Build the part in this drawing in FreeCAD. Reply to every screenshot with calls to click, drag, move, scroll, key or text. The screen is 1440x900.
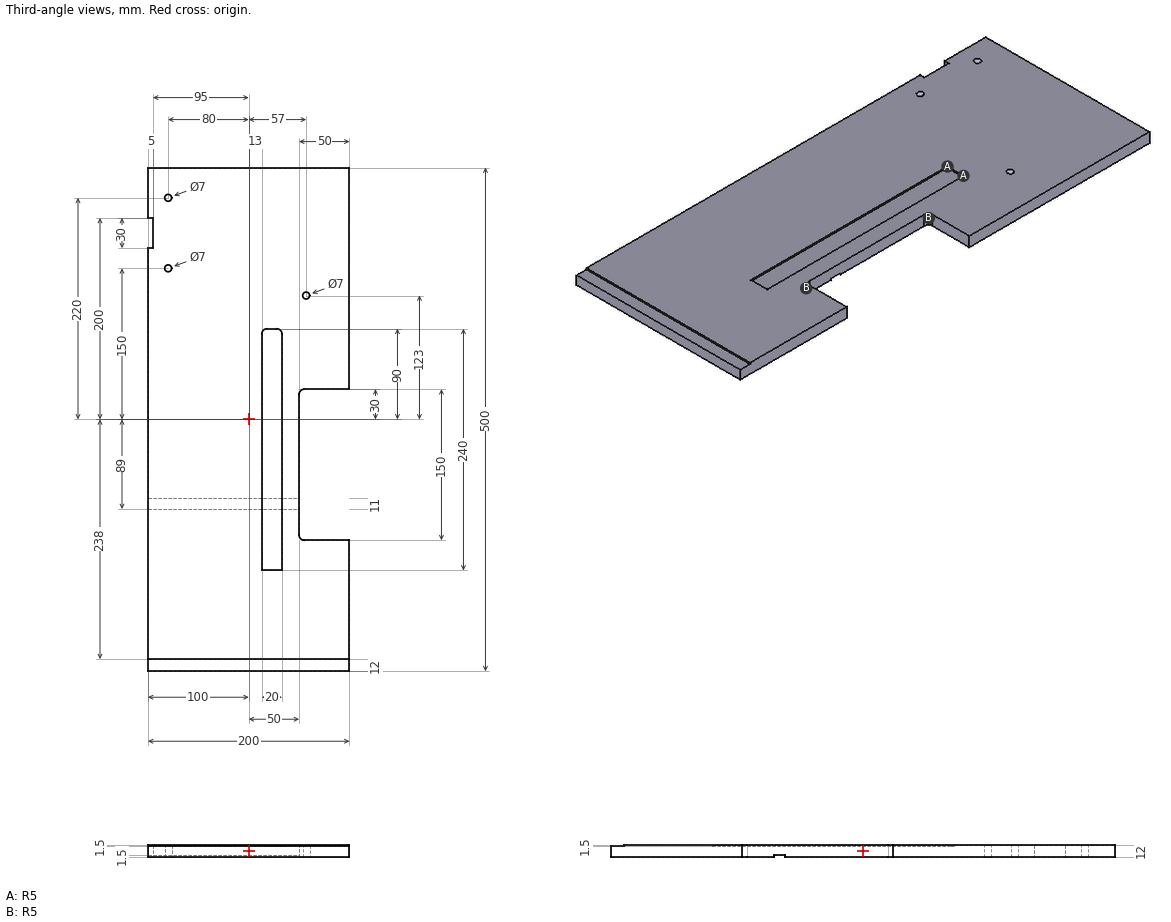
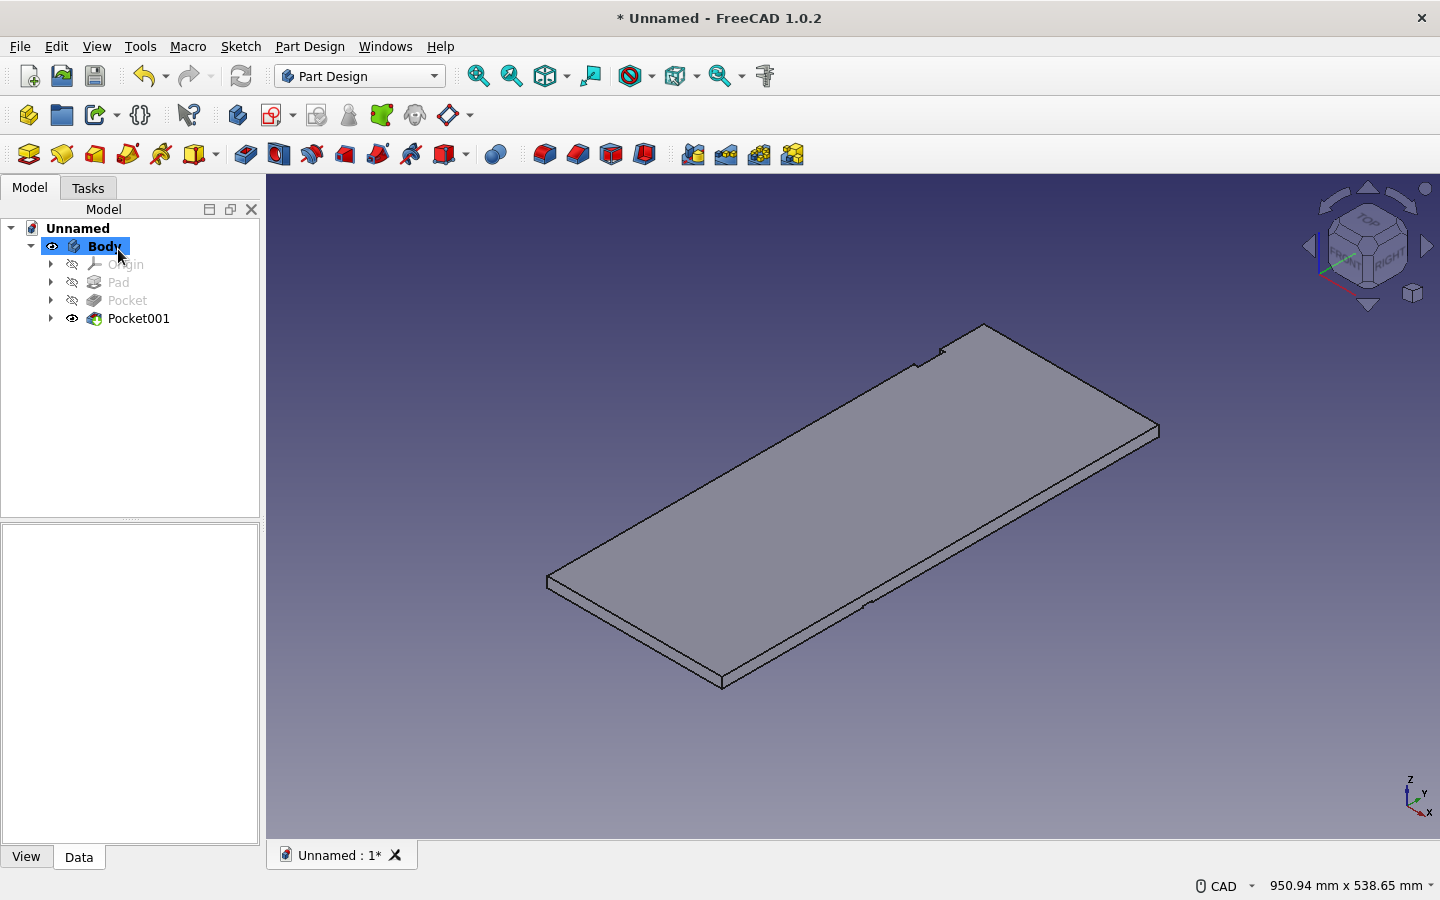
click(915, 463)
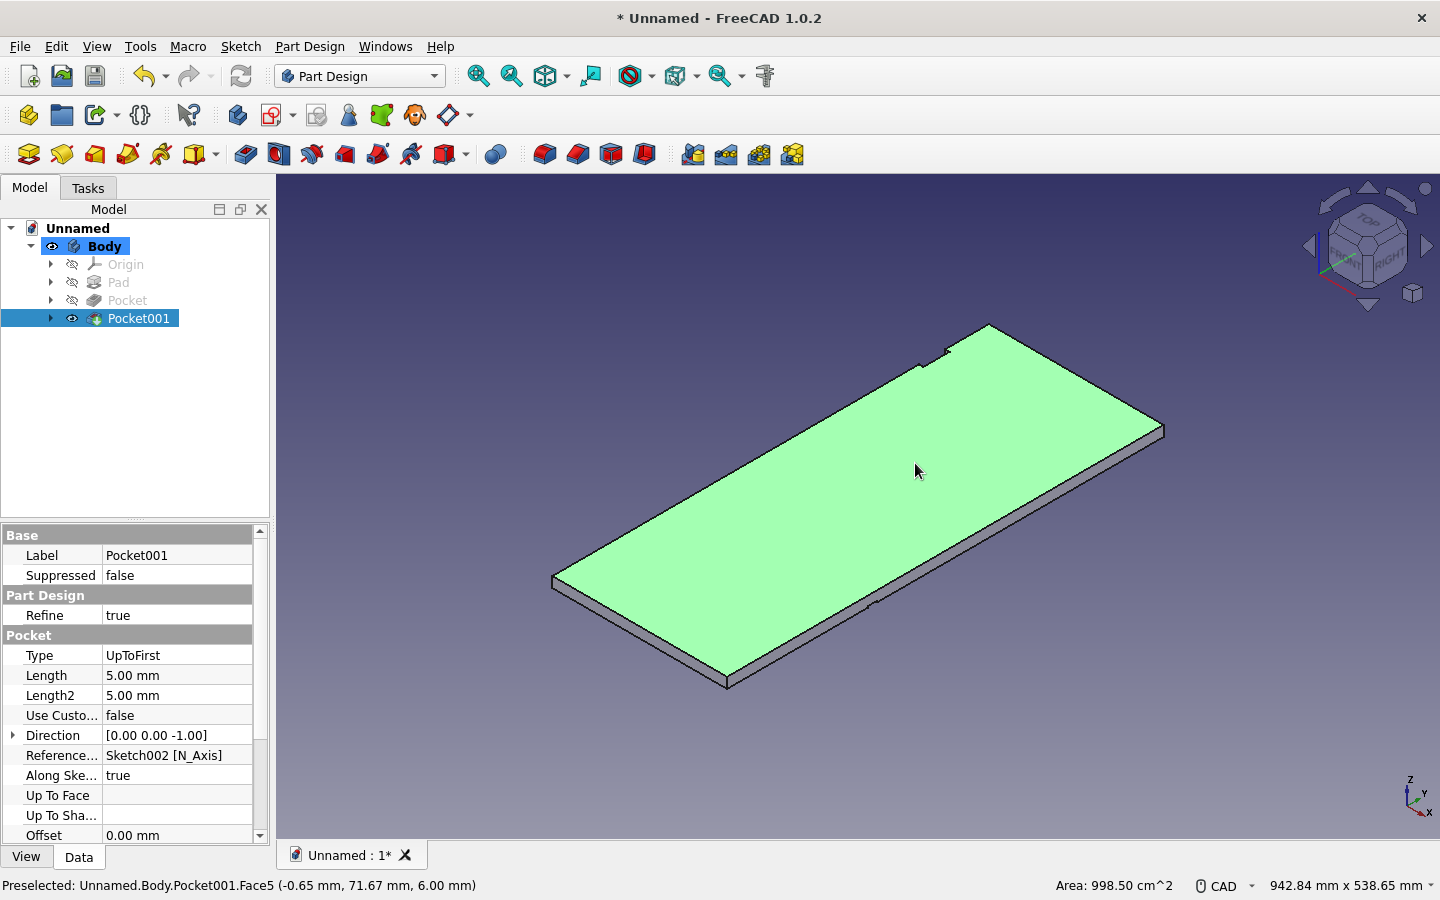
click(270, 116)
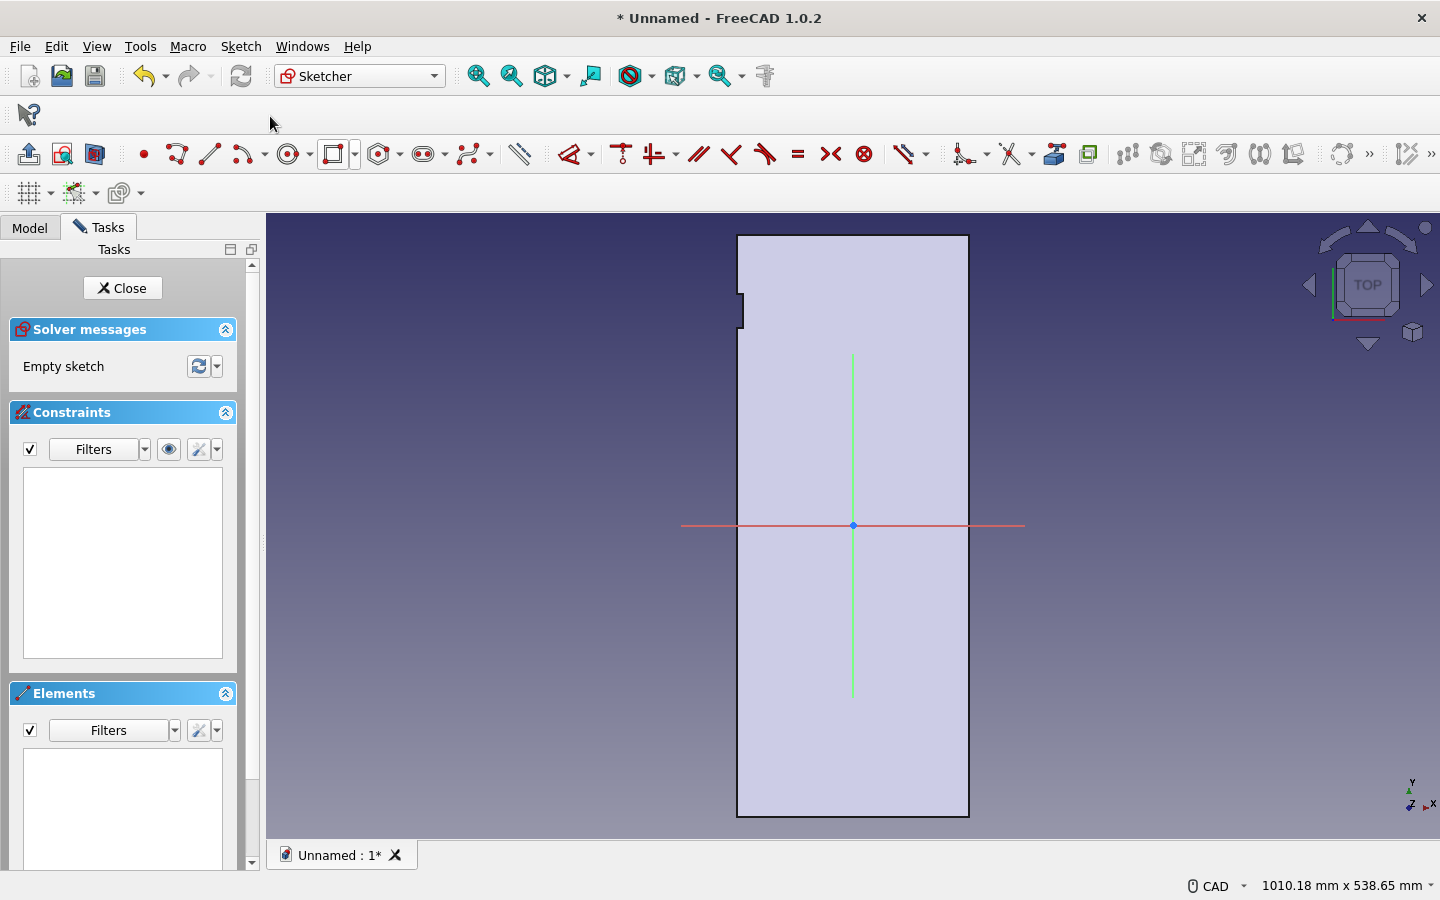
scroll(759, 257, up, 15)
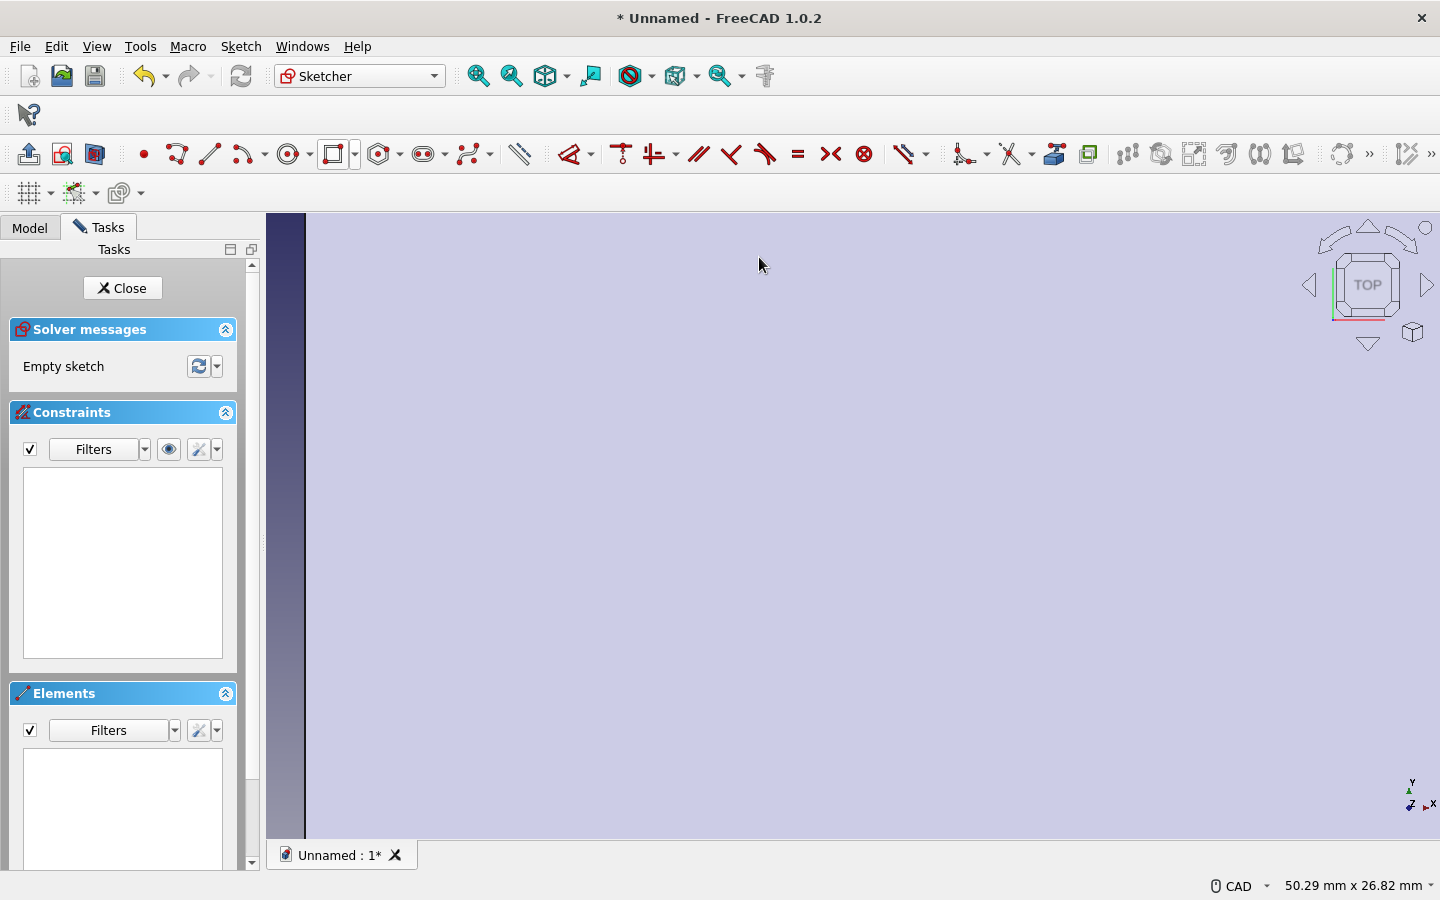
scroll(764, 522, up, 5)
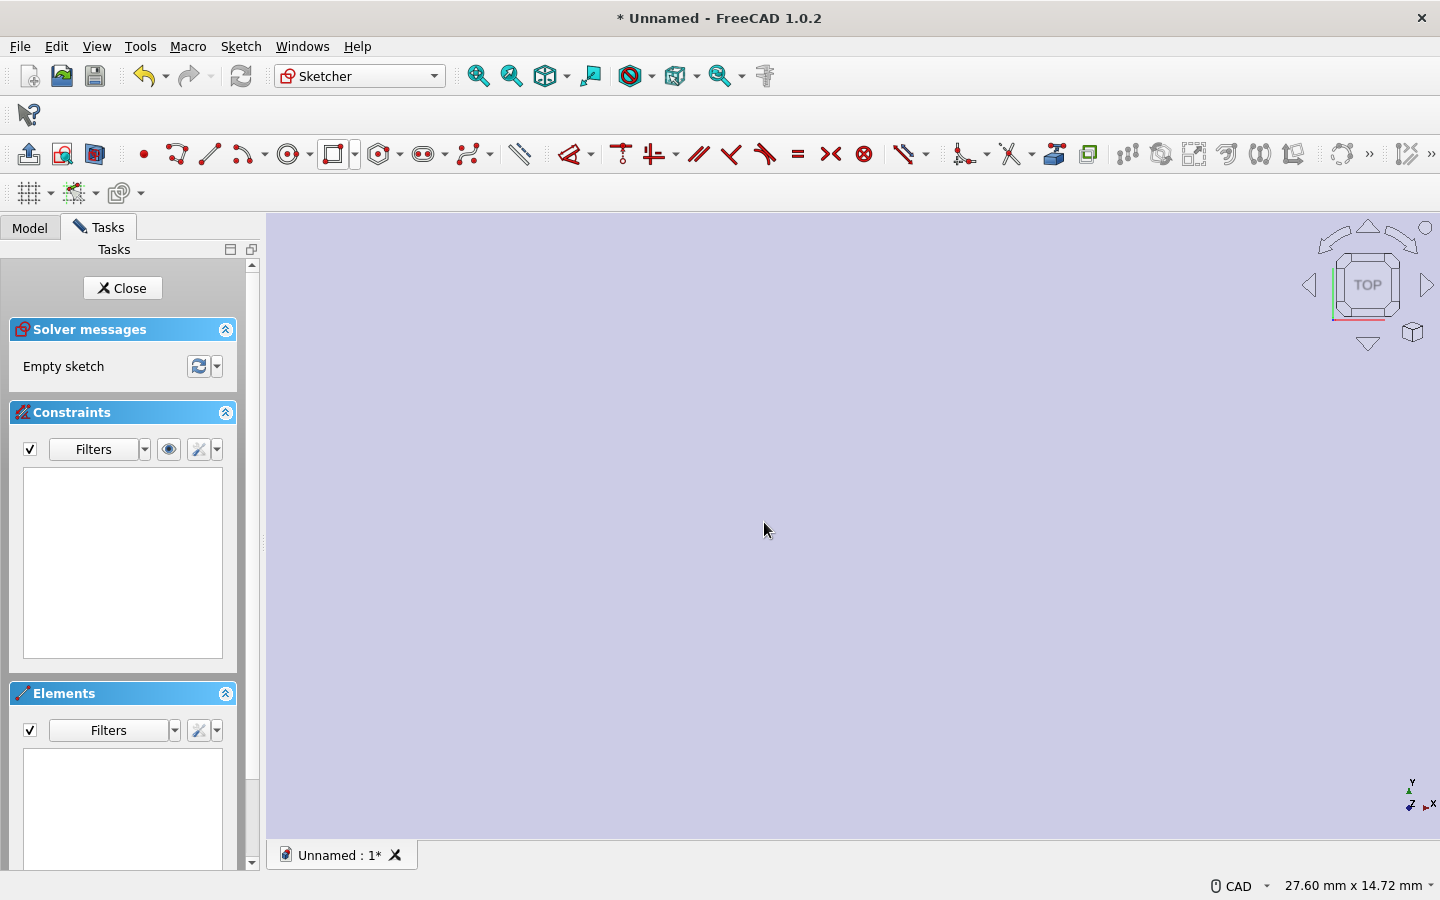
click(288, 154)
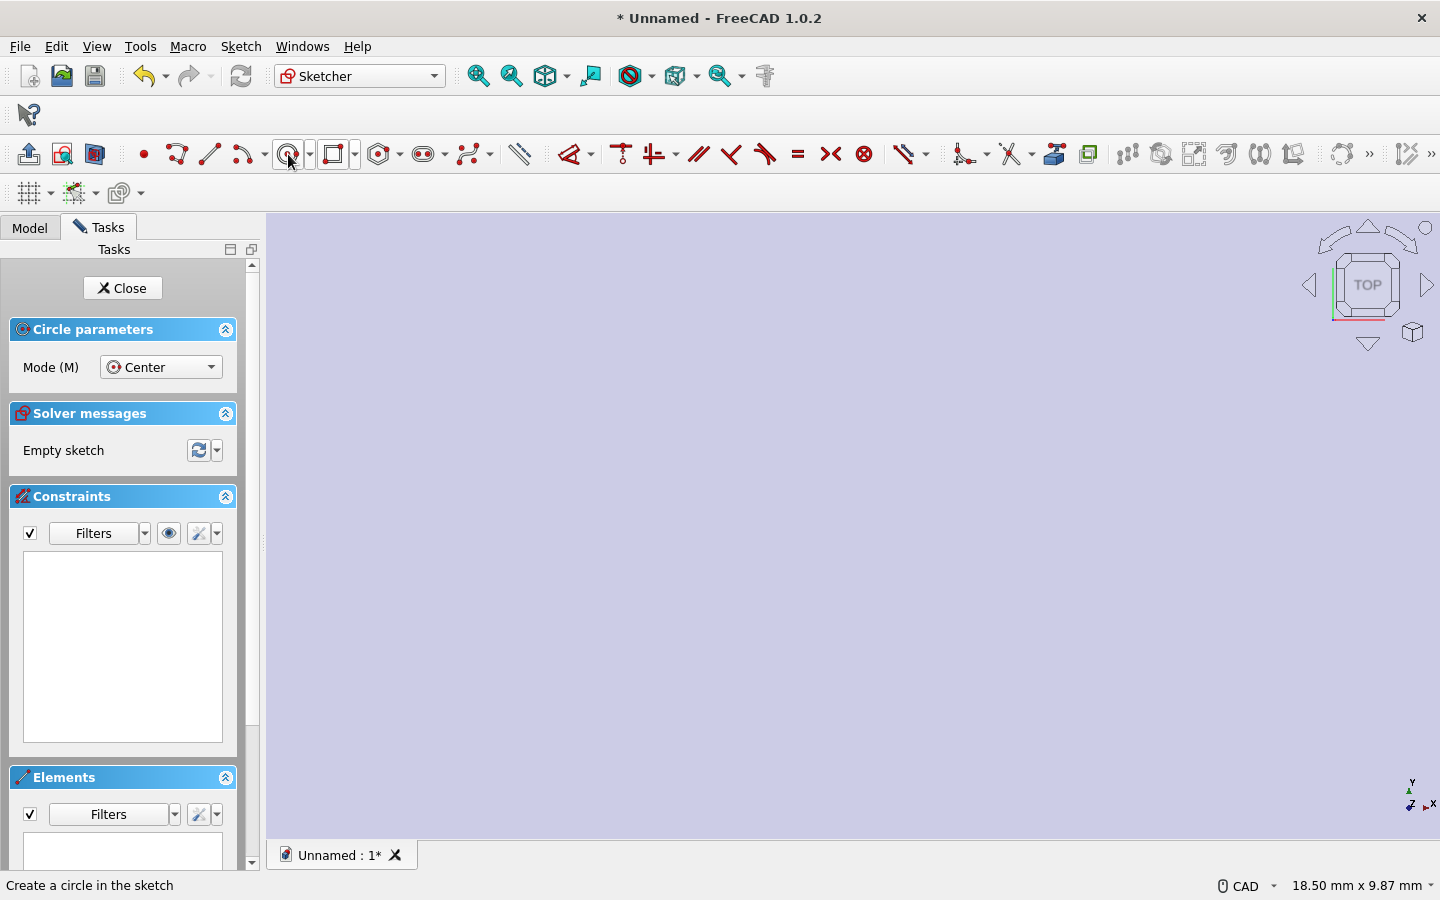
click(784, 525)
move(941, 368)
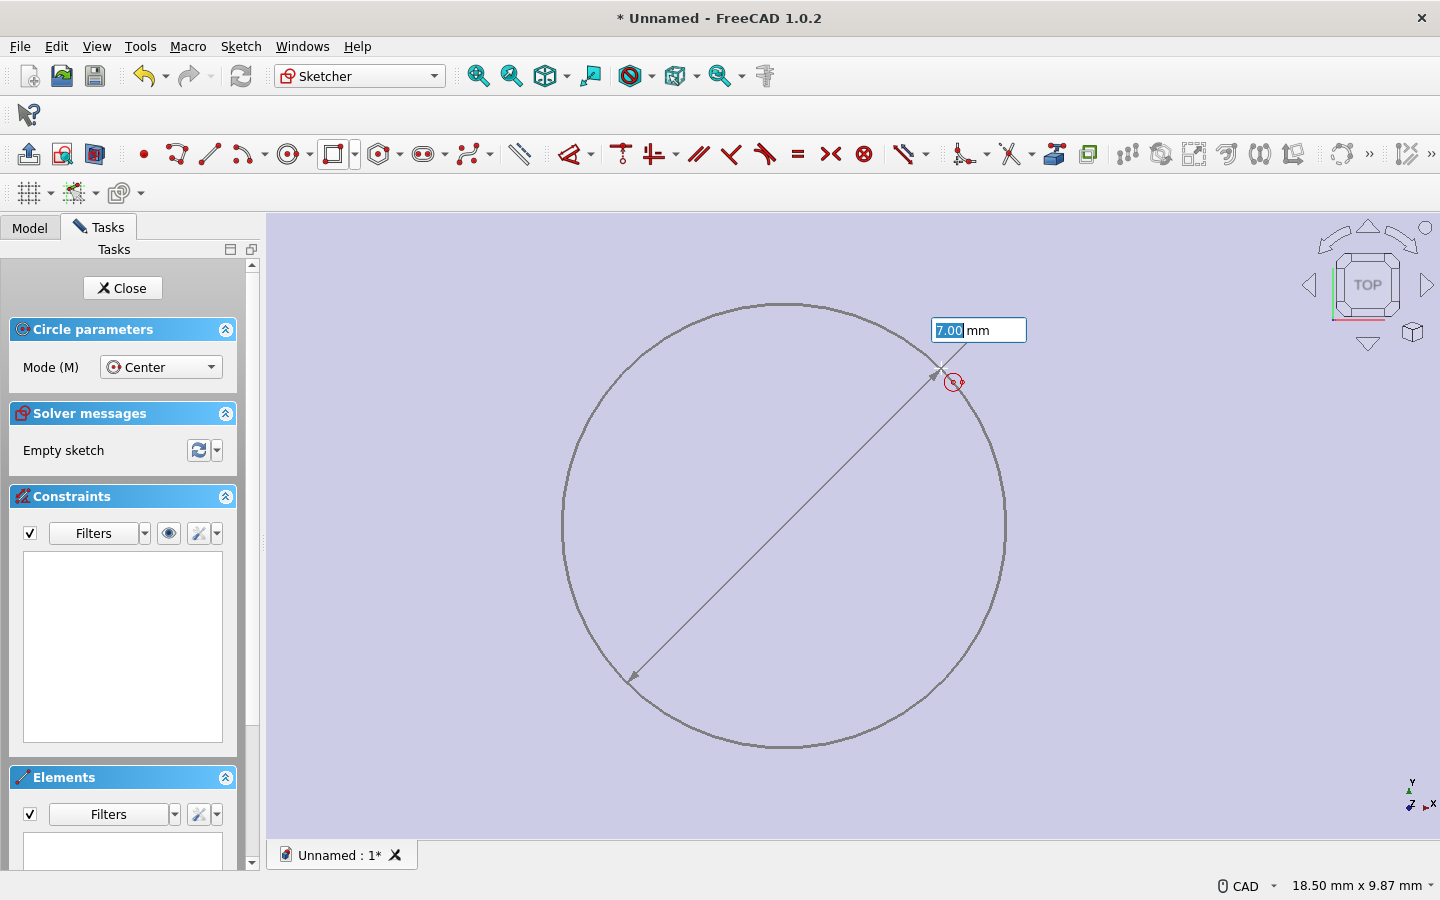
text(7)
key(Return)
key(Escape)